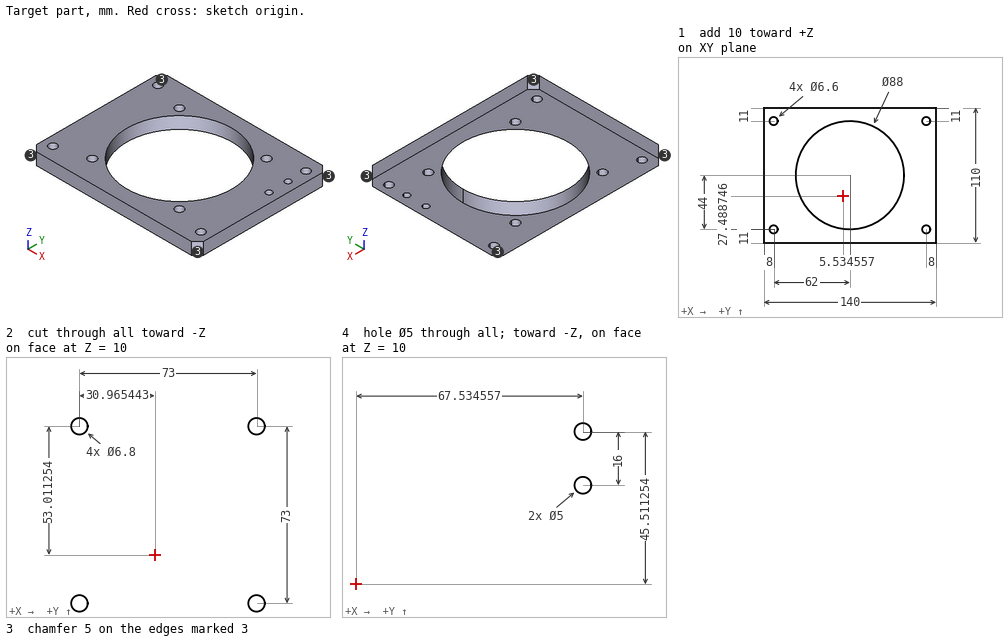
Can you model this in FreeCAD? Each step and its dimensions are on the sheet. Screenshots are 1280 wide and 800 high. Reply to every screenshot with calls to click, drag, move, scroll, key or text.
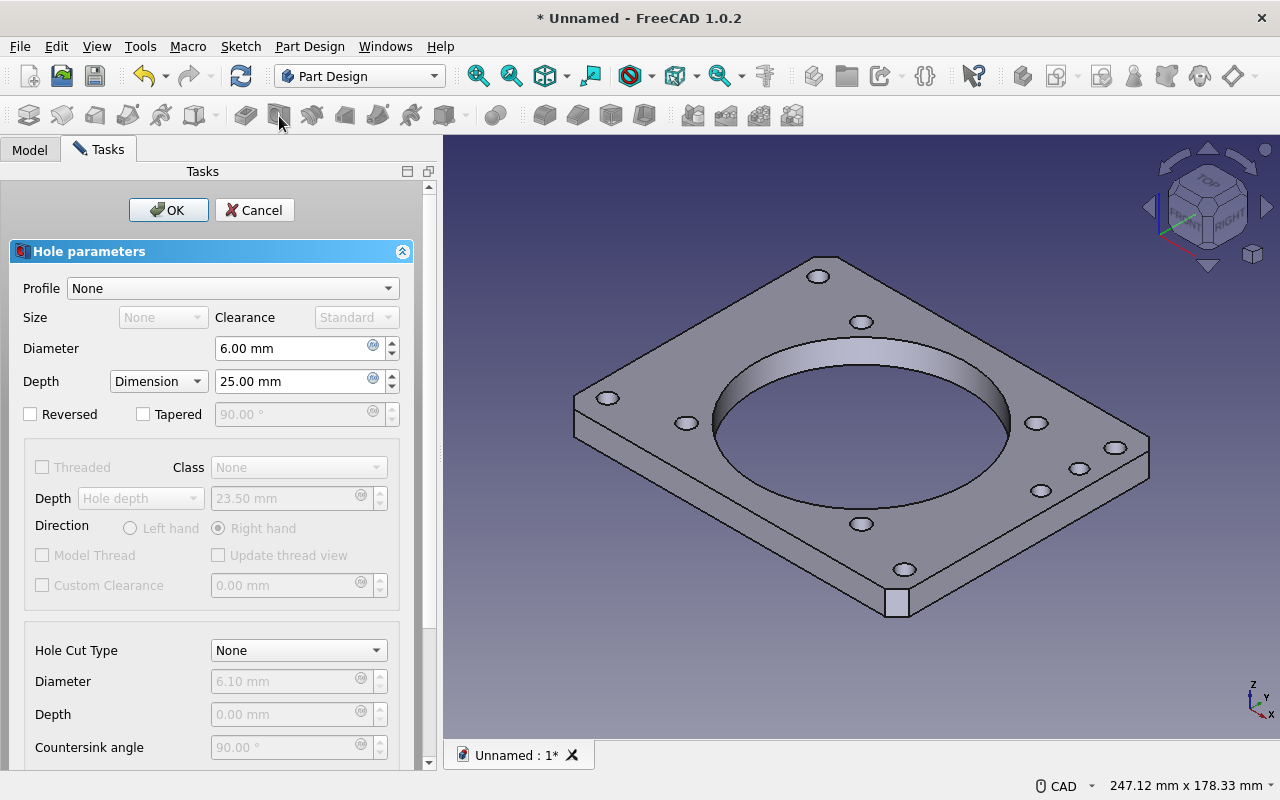
triple_click(300, 348)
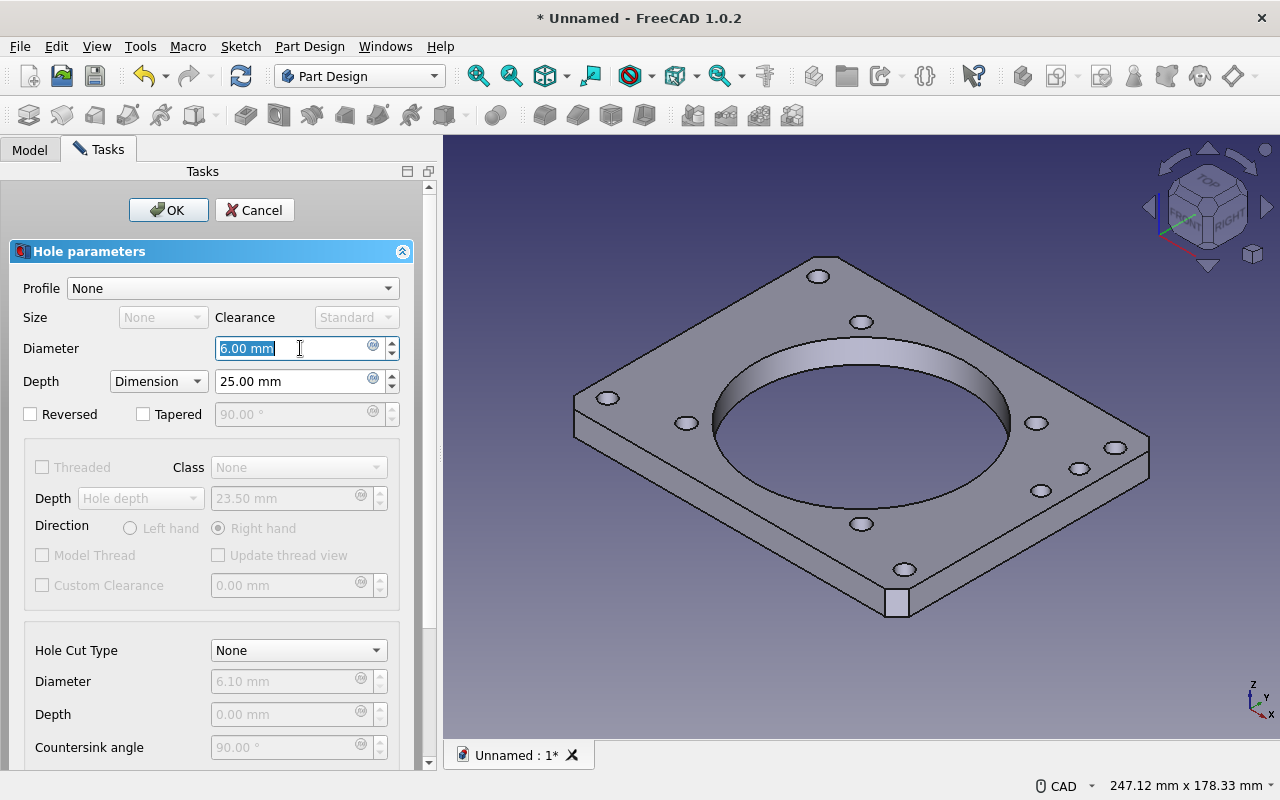
text(5)
key(Tab)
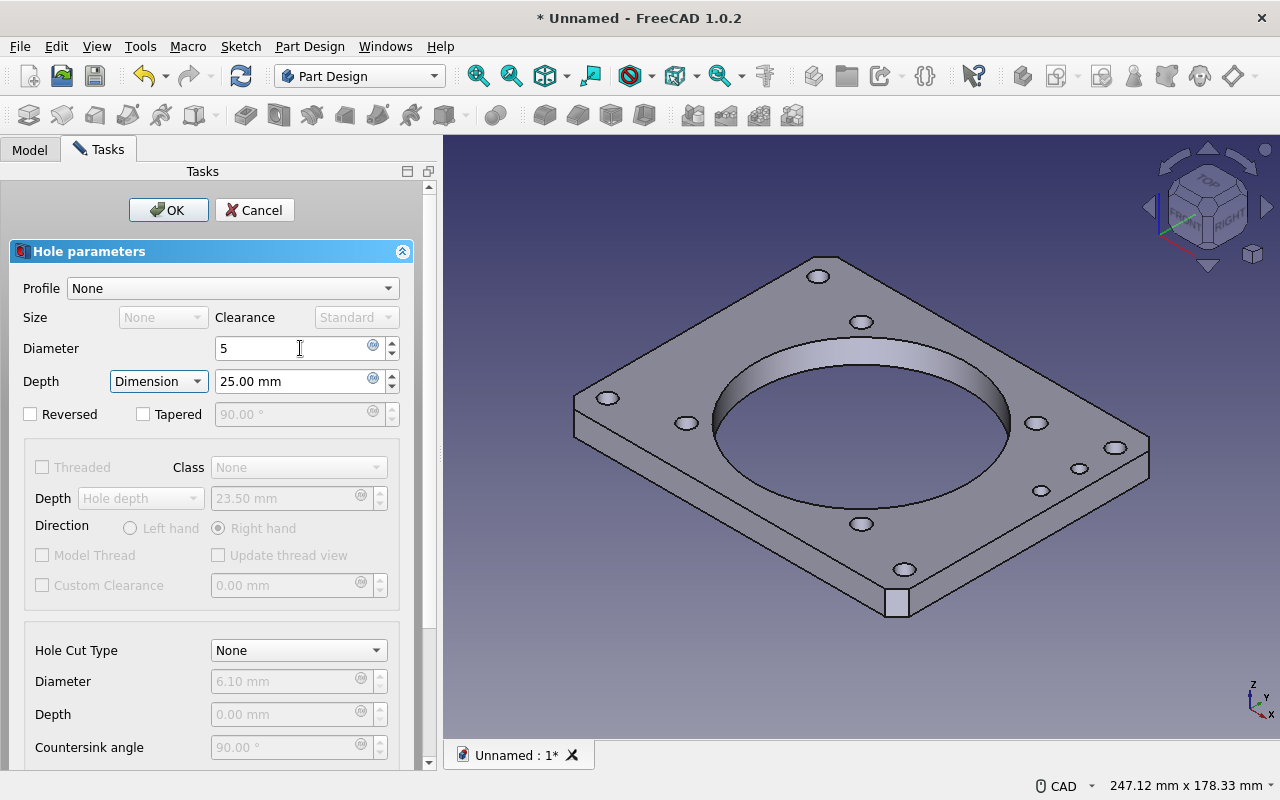
click(160, 382)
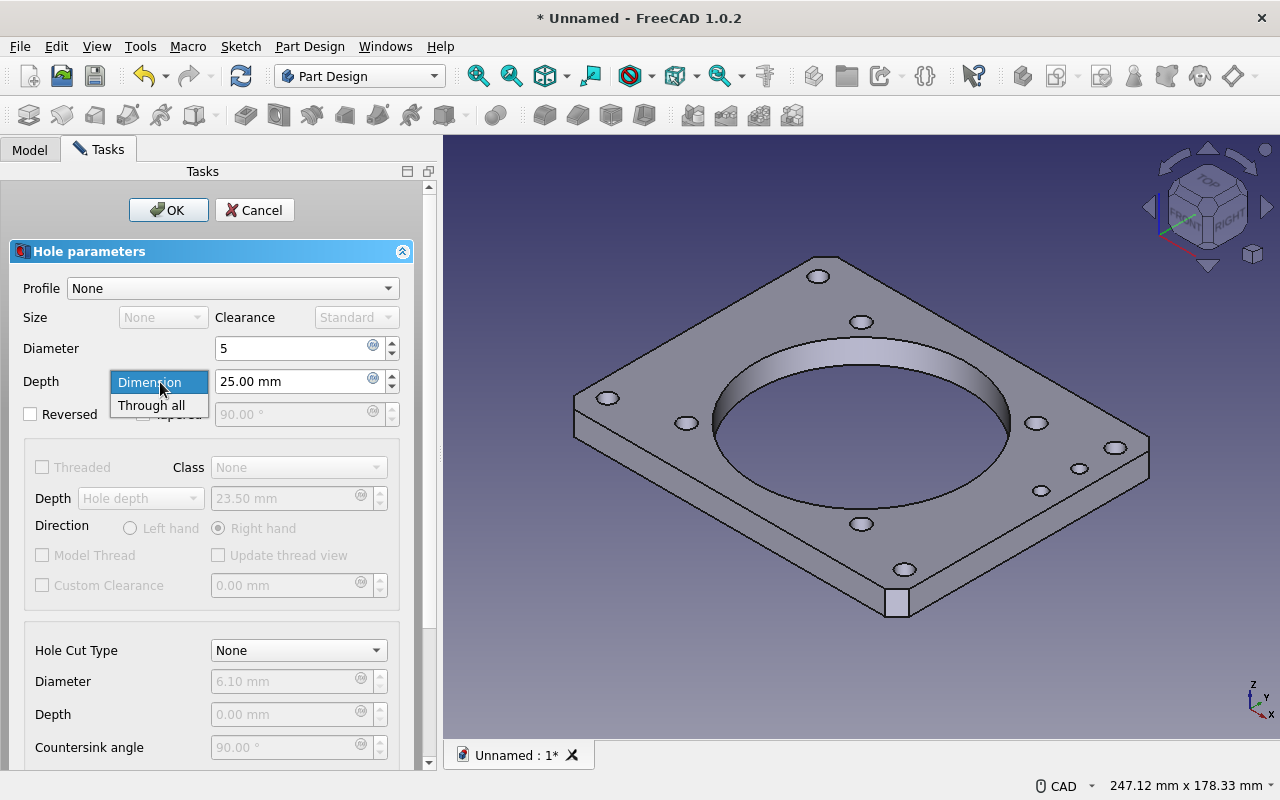
click(158, 406)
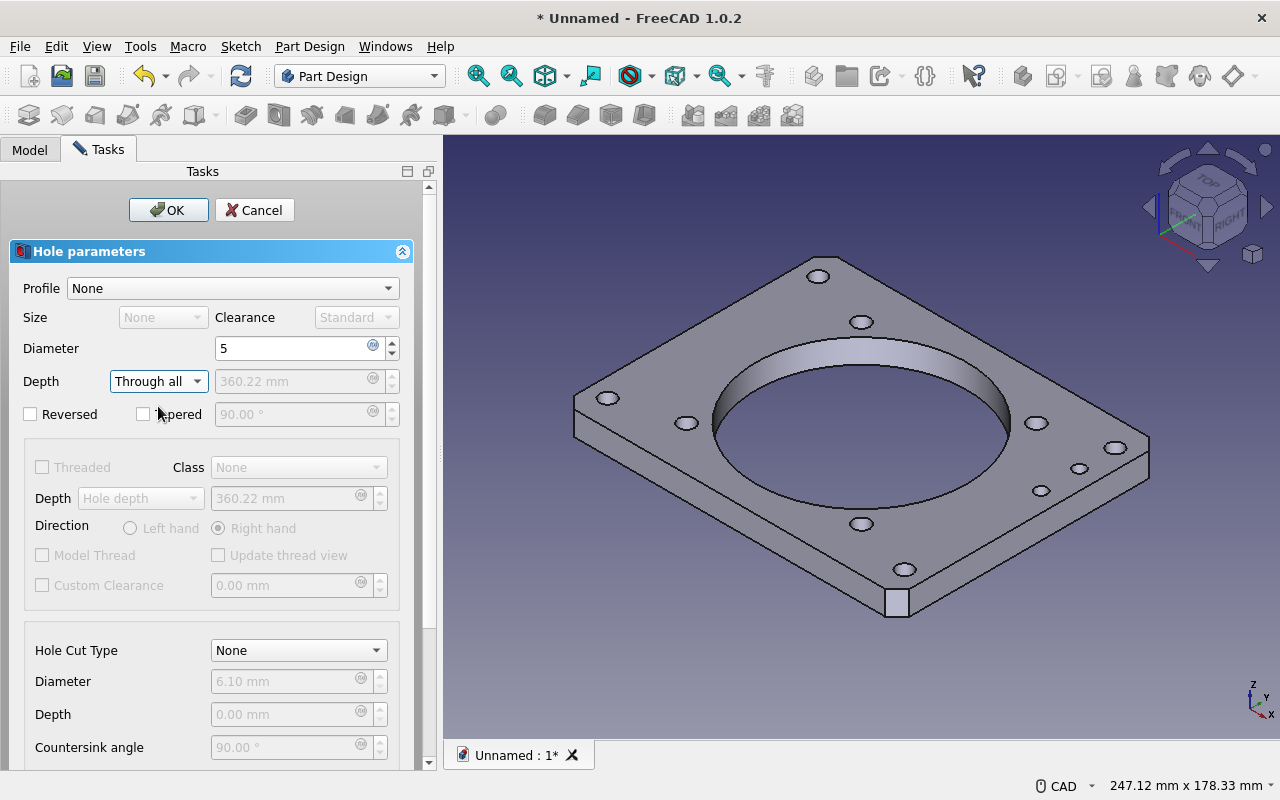
click(169, 210)